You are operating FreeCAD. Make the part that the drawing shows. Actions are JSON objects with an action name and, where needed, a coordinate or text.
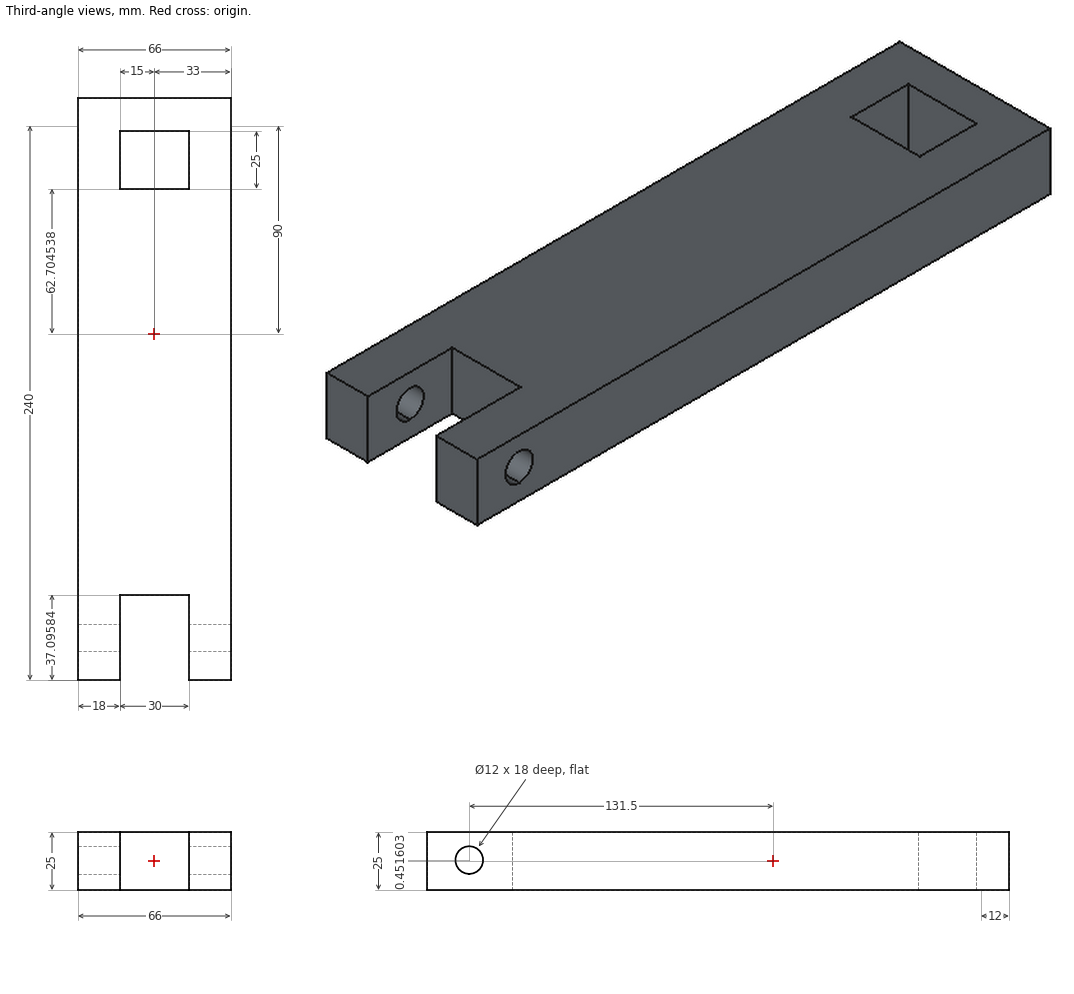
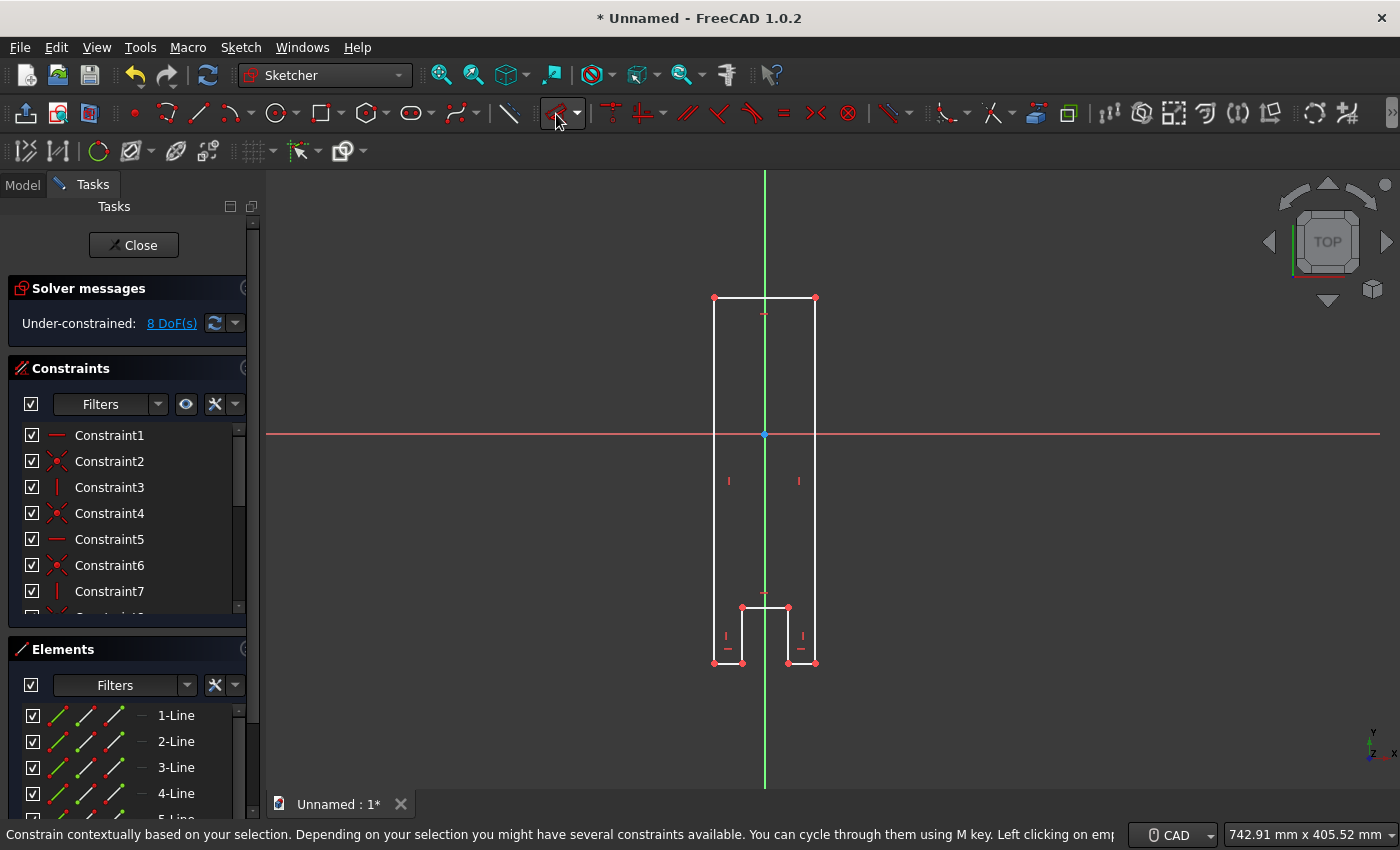
{"action": "left_click", "coordinate": [785, 298]}
{"action": "left_click", "coordinate": [741, 264]}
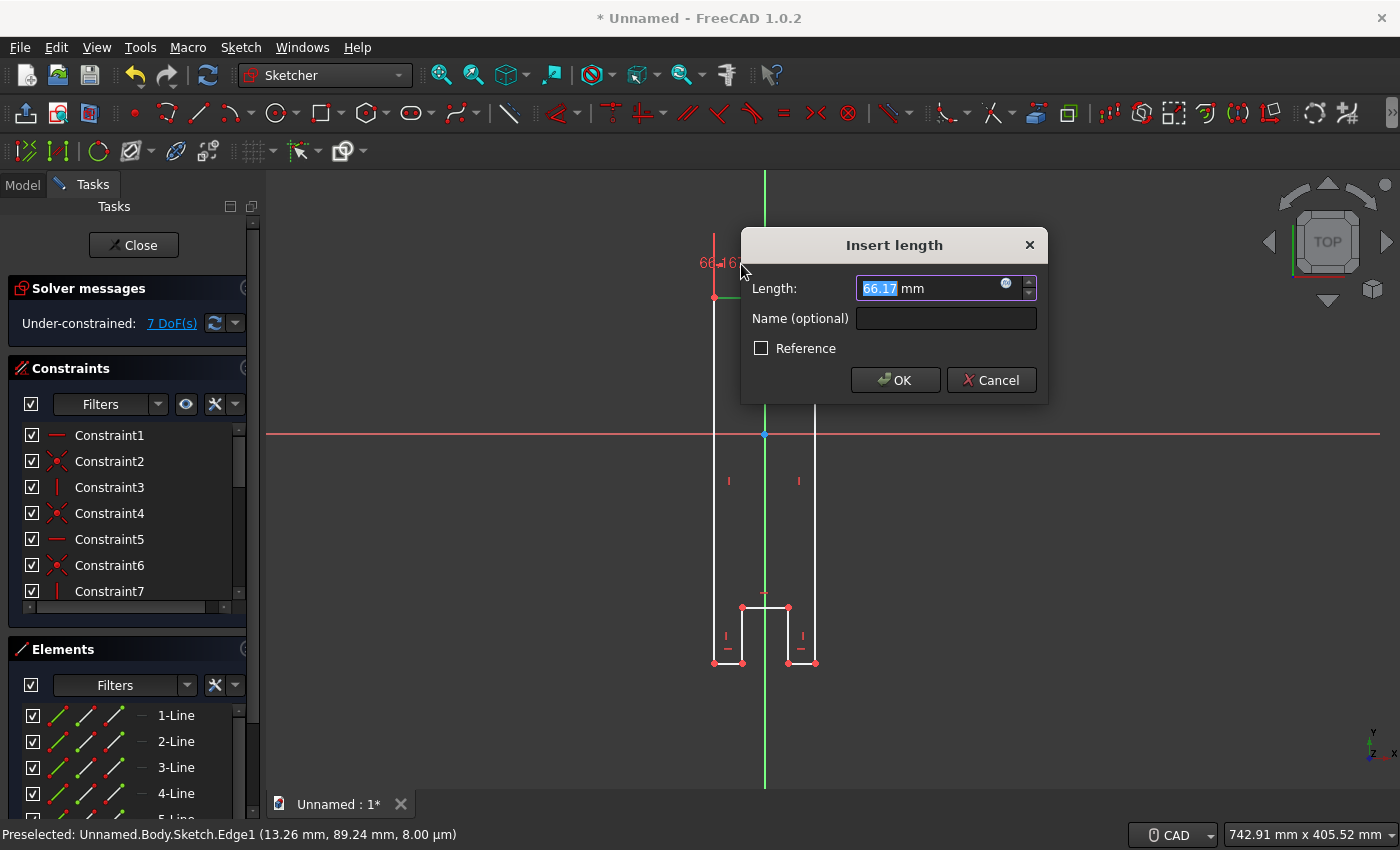
{"action": "type", "text": "66"}
{"action": "key", "text": "Return"}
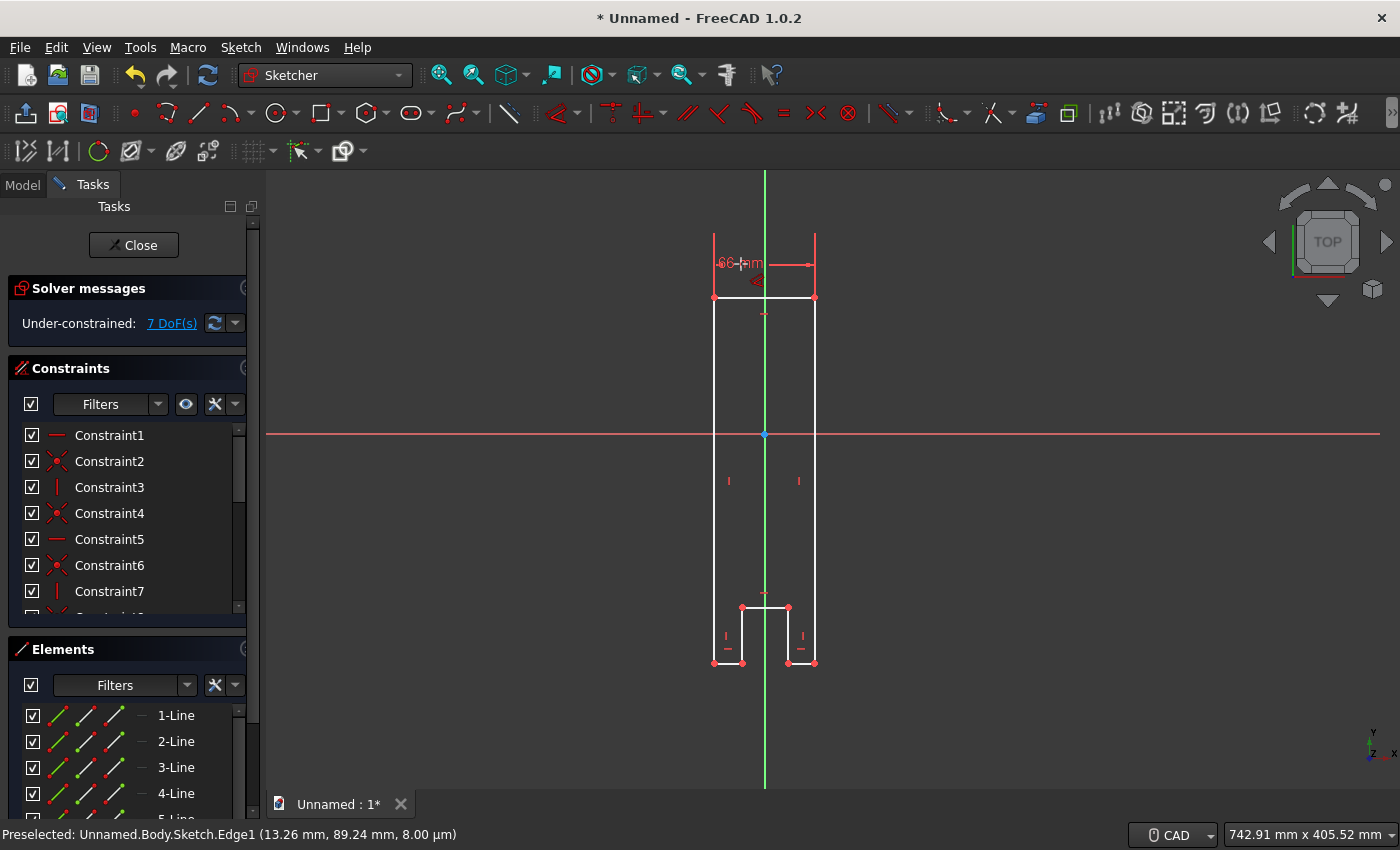
{"action": "scroll", "coordinate": [725, 664], "scroll_direction": "up", "scroll_amount": 2}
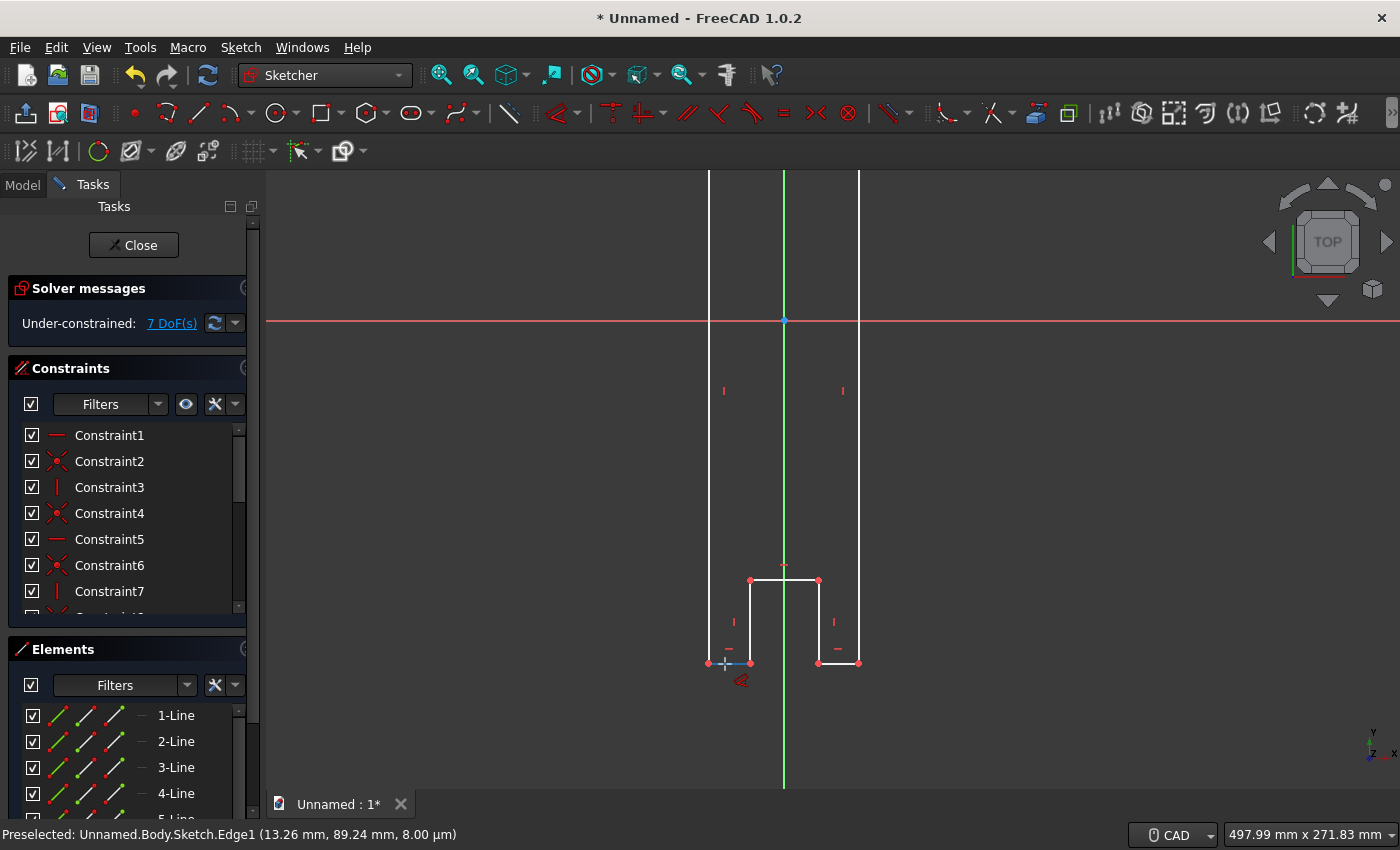
{"action": "left_click", "coordinate": [725, 664]}
{"action": "left_click", "coordinate": [729, 698]}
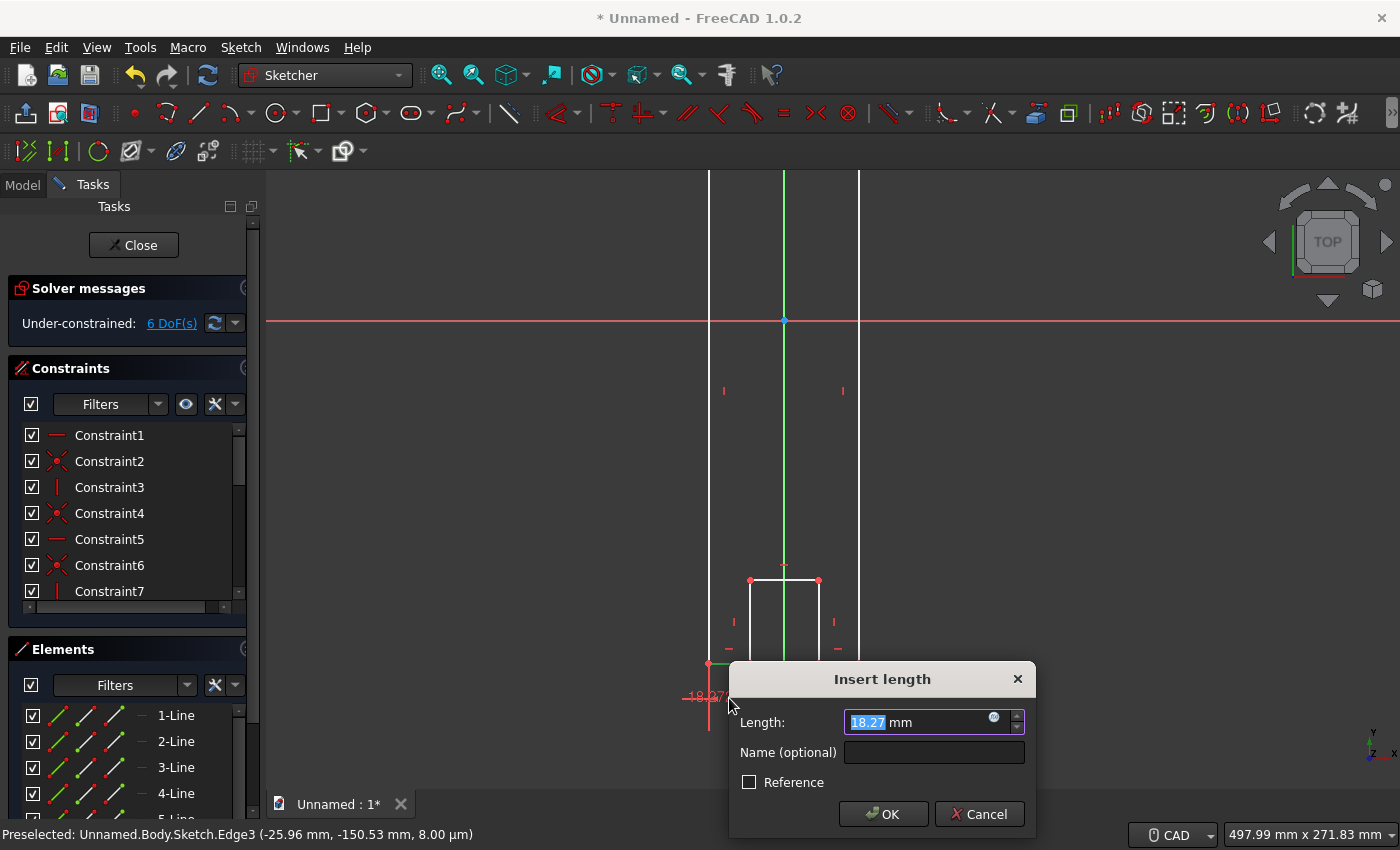
{"action": "type", "text": "18"}
{"action": "key", "text": "Return"}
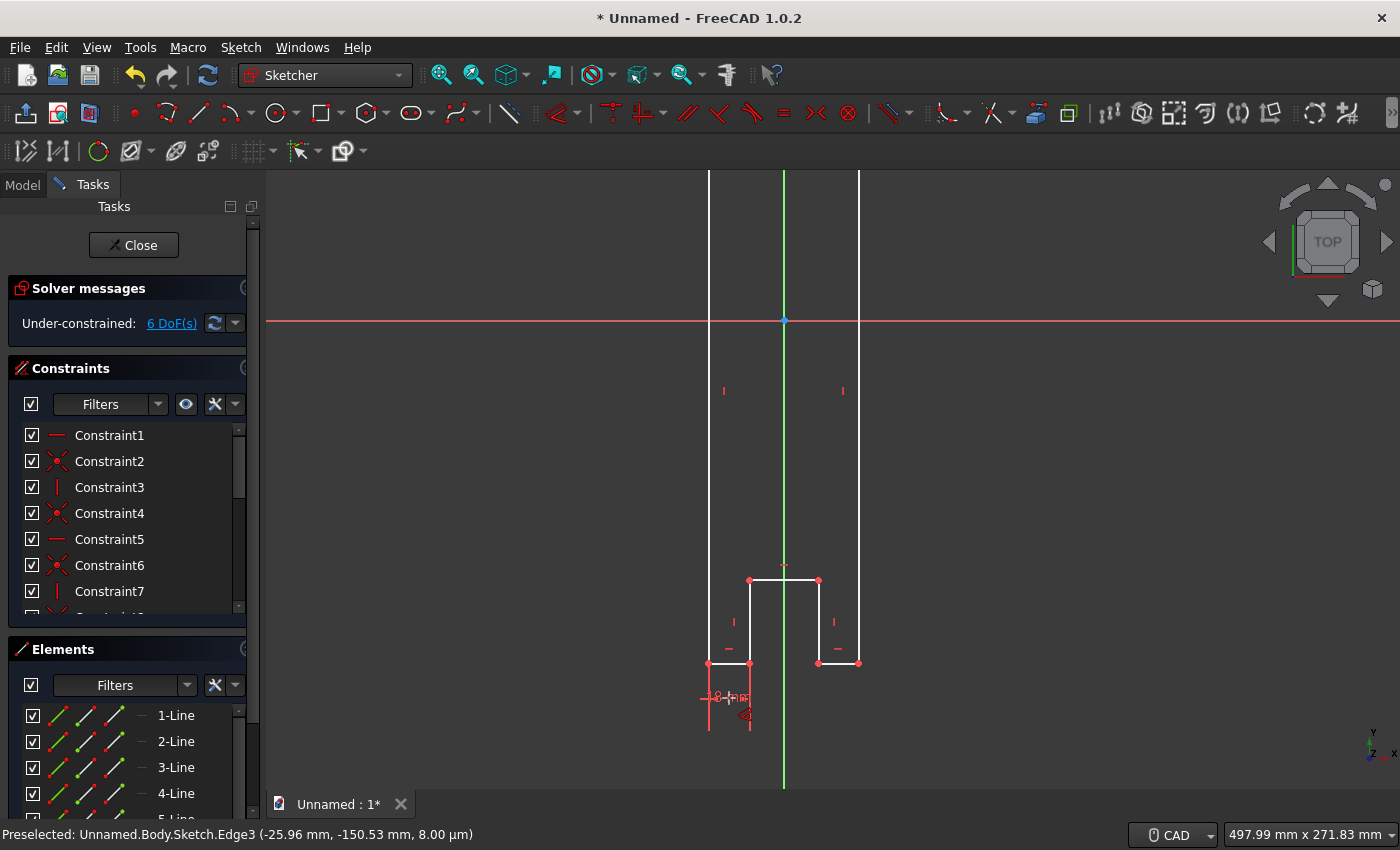
{"action": "left_click", "coordinate": [770, 580]}
{"action": "left_click", "coordinate": [768, 614]}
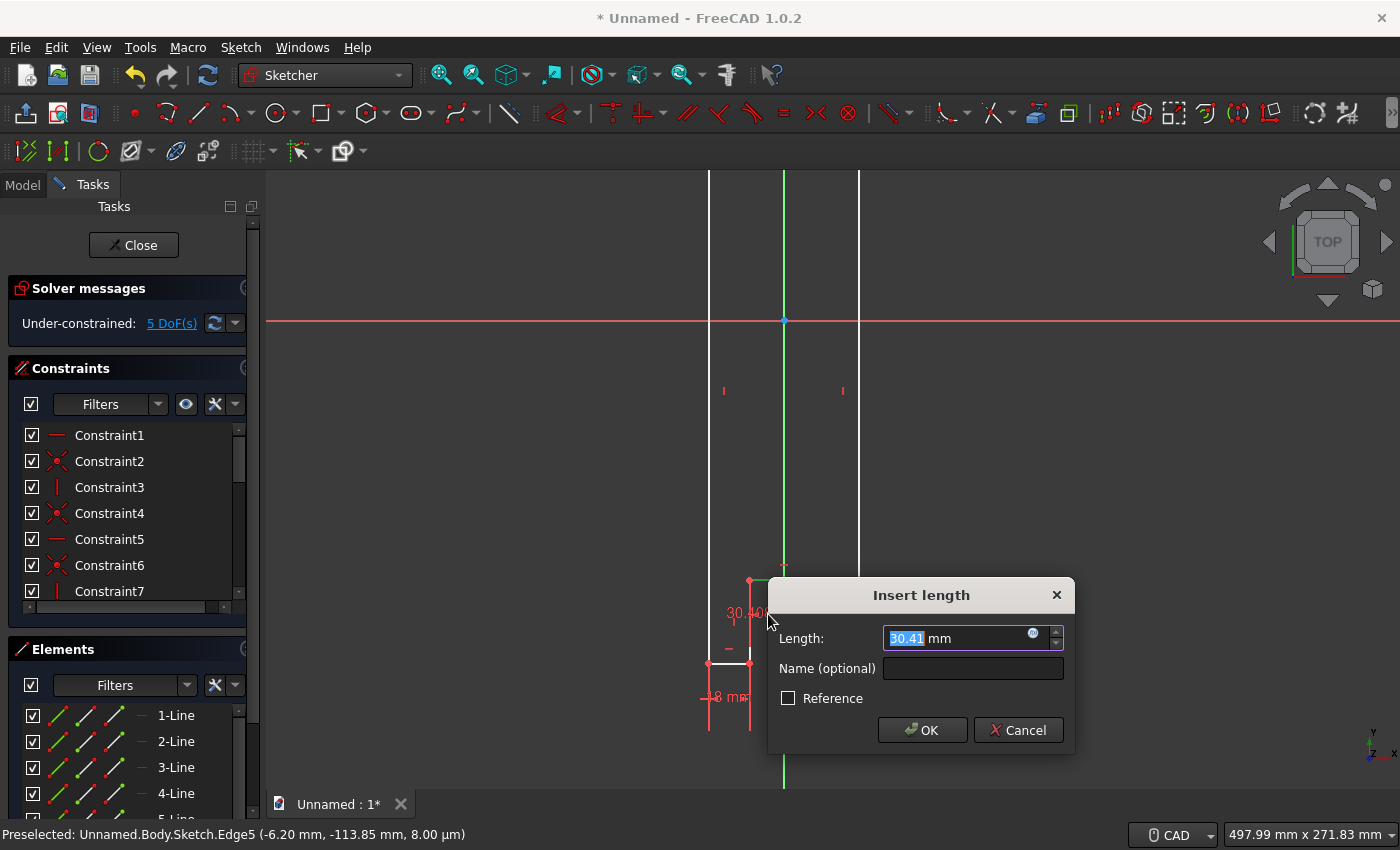
{"action": "type", "text": "30"}
{"action": "key", "text": "Return"}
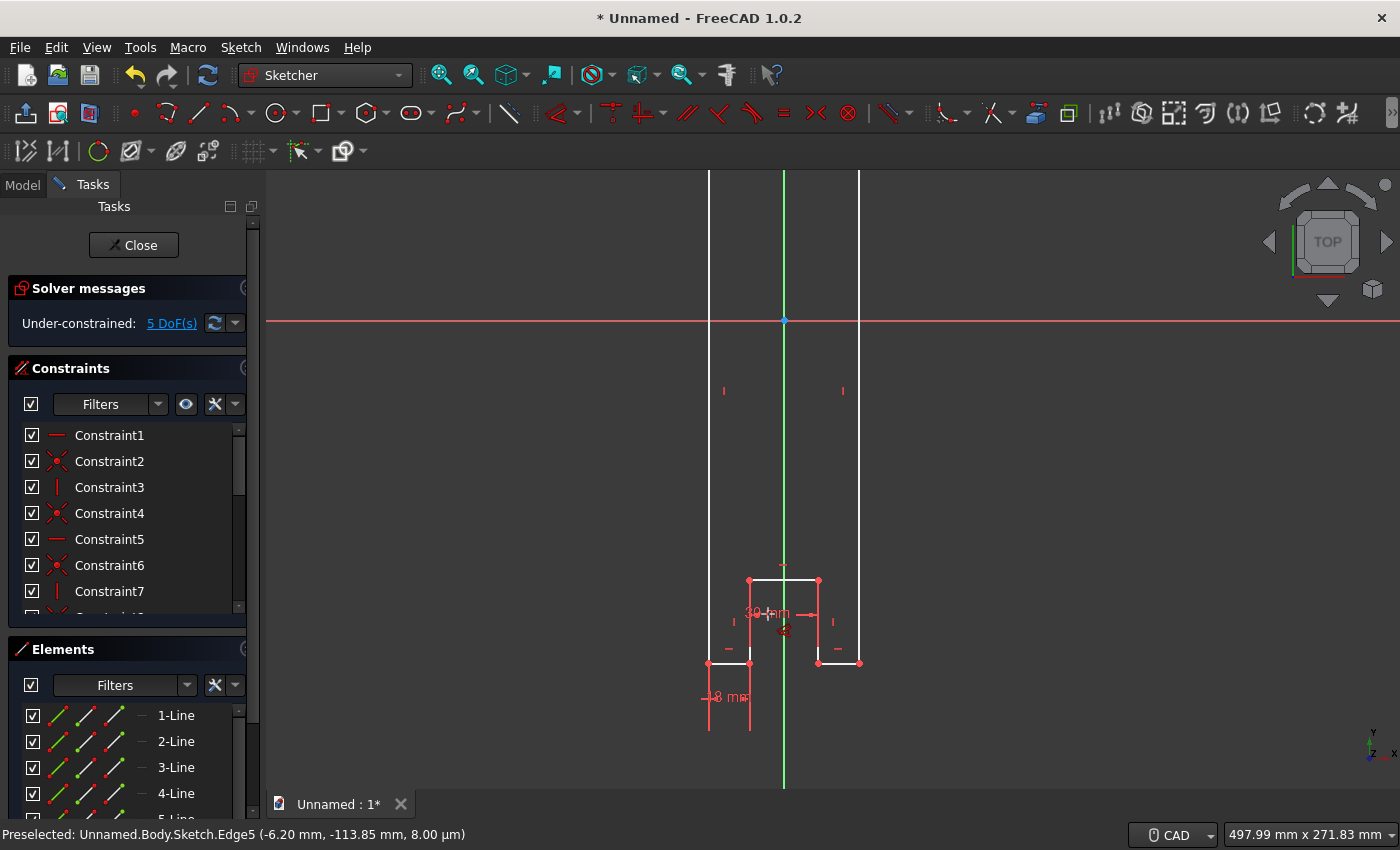
{"action": "left_click", "coordinate": [709, 281]}
{"action": "left_click", "coordinate": [675, 431]}